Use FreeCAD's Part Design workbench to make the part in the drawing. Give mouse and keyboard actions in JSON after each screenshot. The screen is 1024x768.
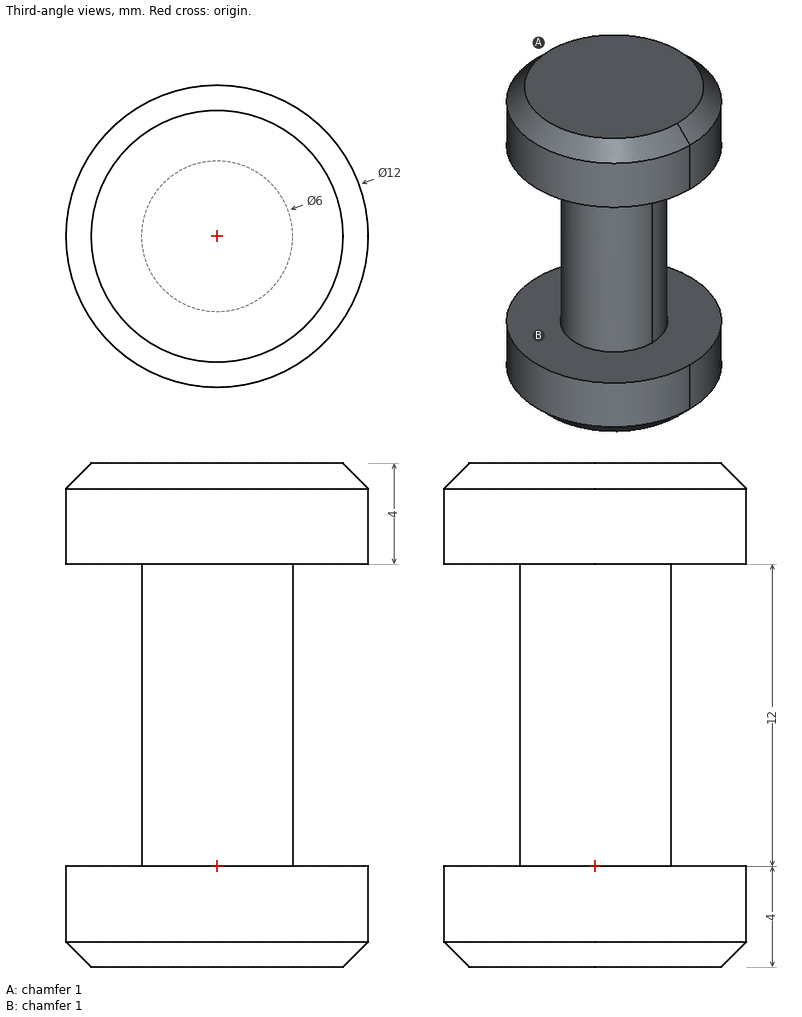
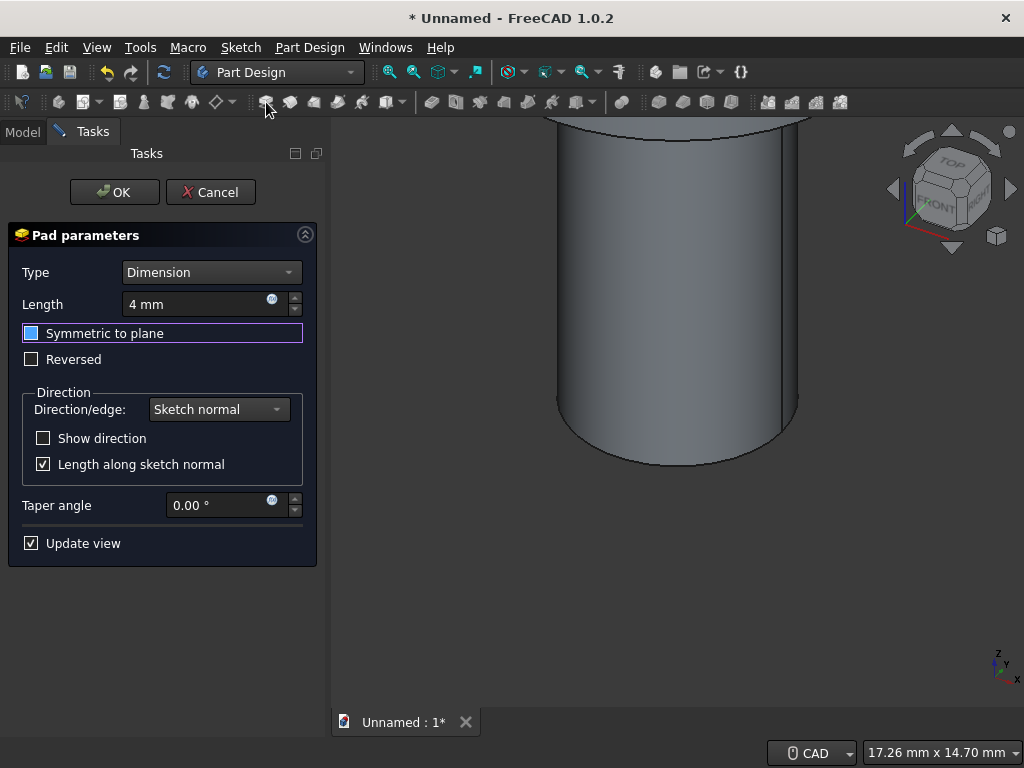
{"action": "left_click", "coordinate": [115, 192]}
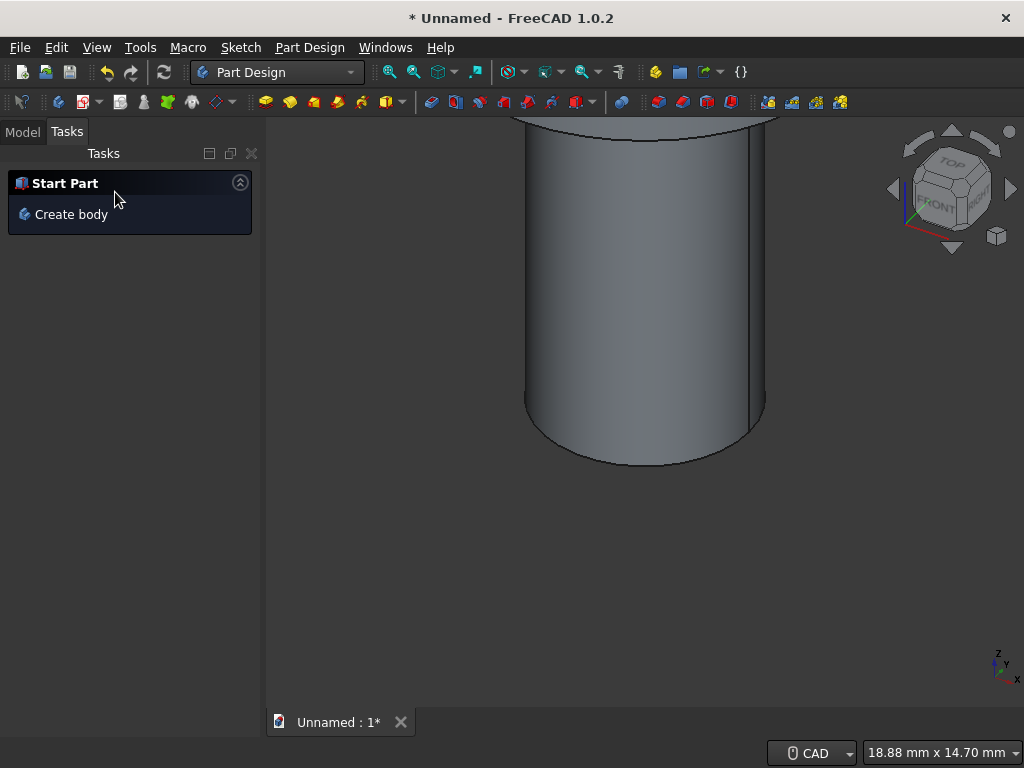
{"action": "left_click", "coordinate": [390, 72]}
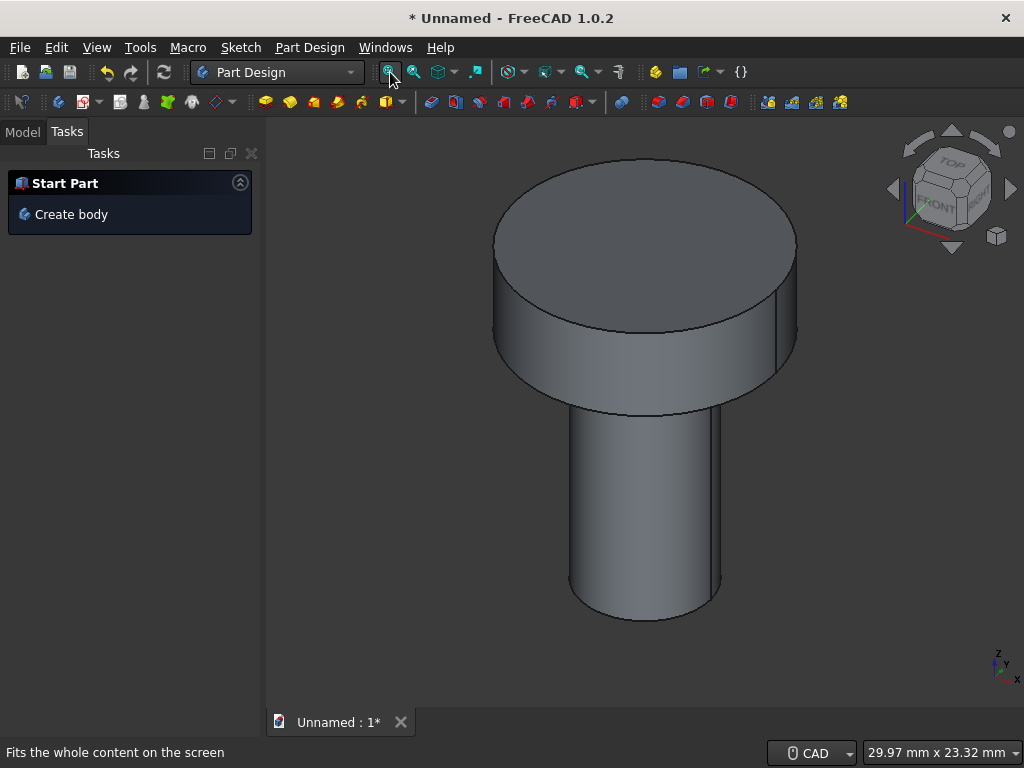
{"action": "left_click", "coordinate": [494, 254]}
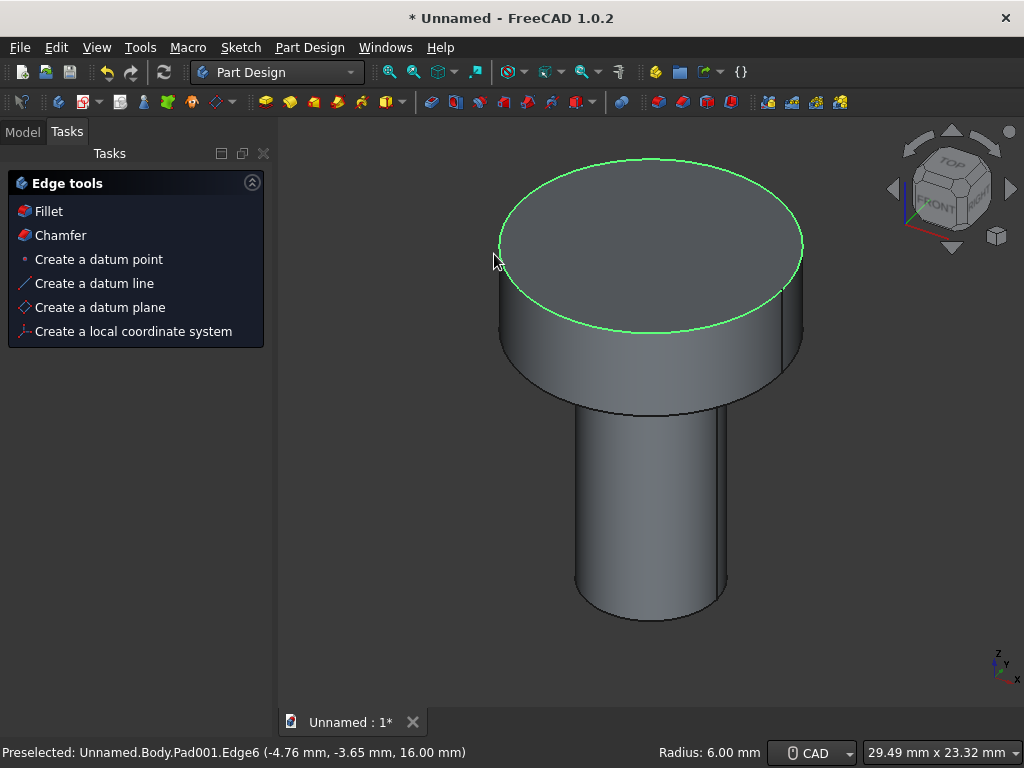
{"action": "left_click", "coordinate": [684, 102]}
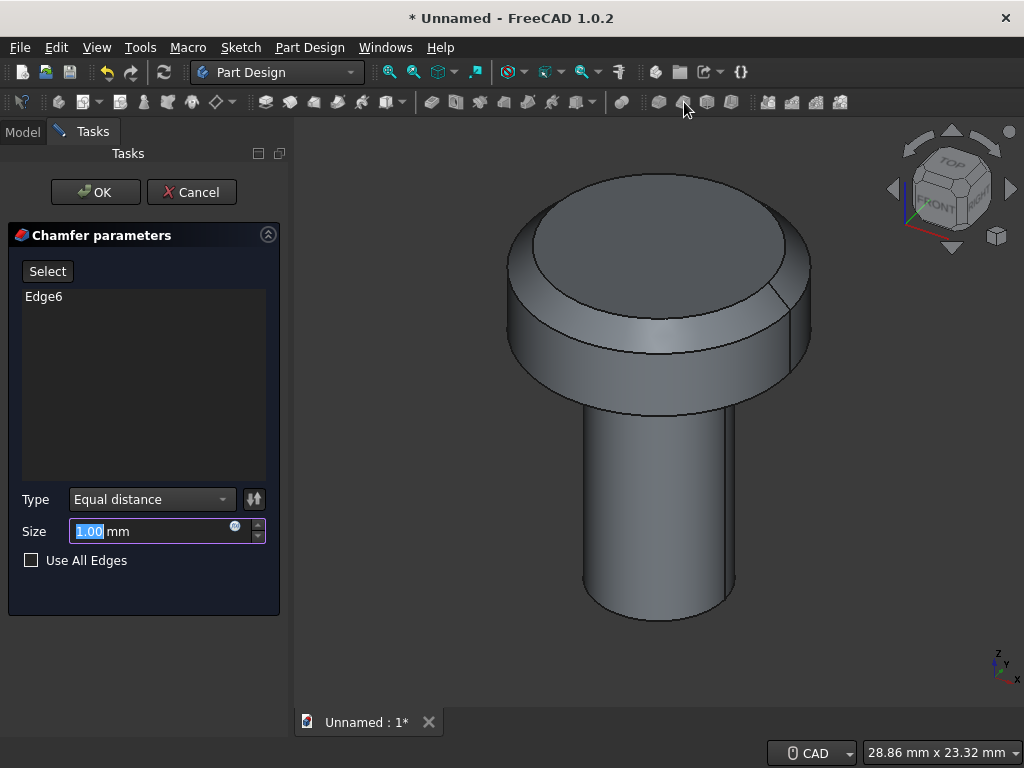
{"action": "type", "text": "1"}
{"action": "key", "text": "Tab"}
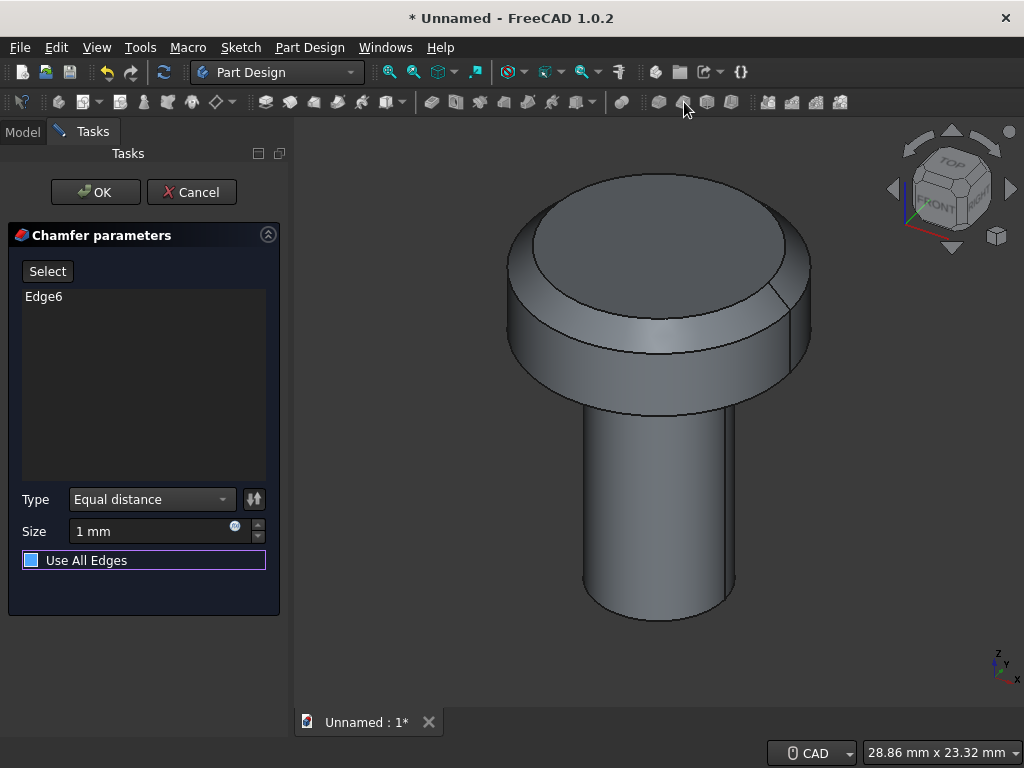
{"action": "left_click", "coordinate": [96, 192]}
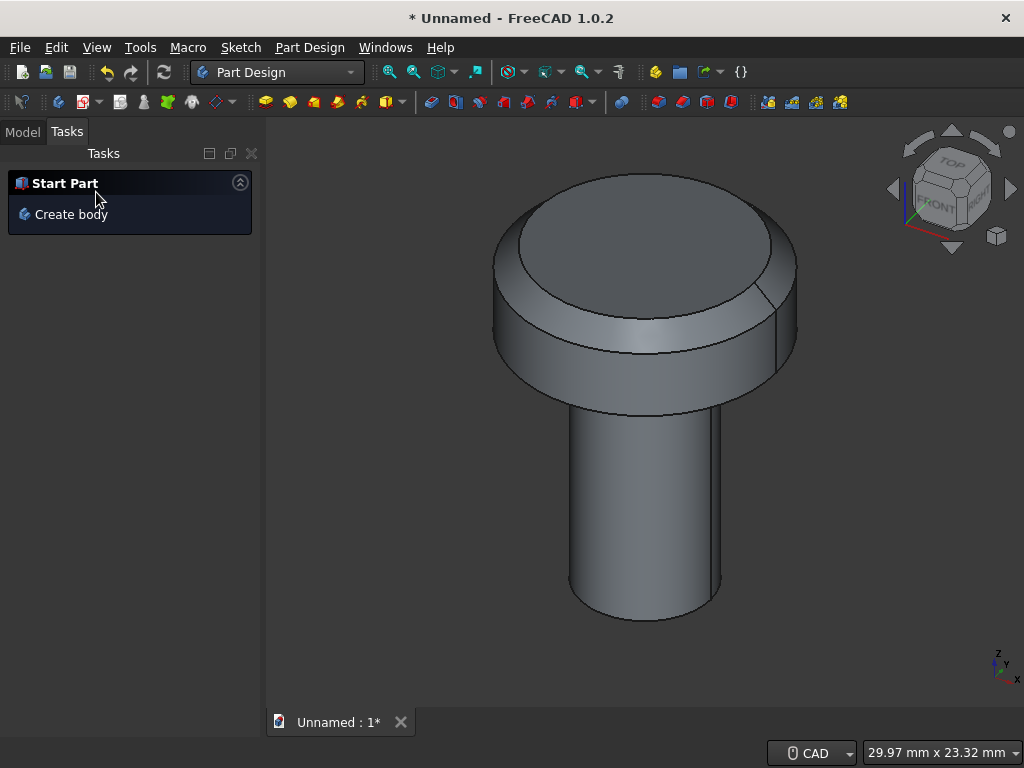
{"action": "left_click", "coordinate": [23, 131]}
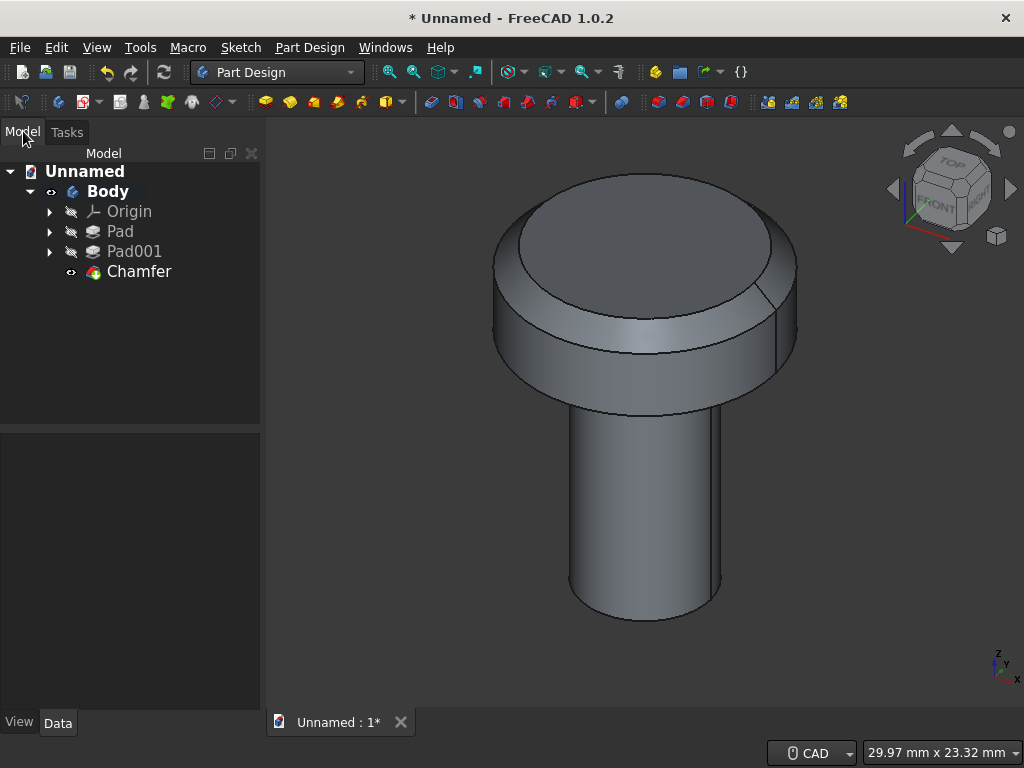
{"action": "left_click", "coordinate": [50, 212]}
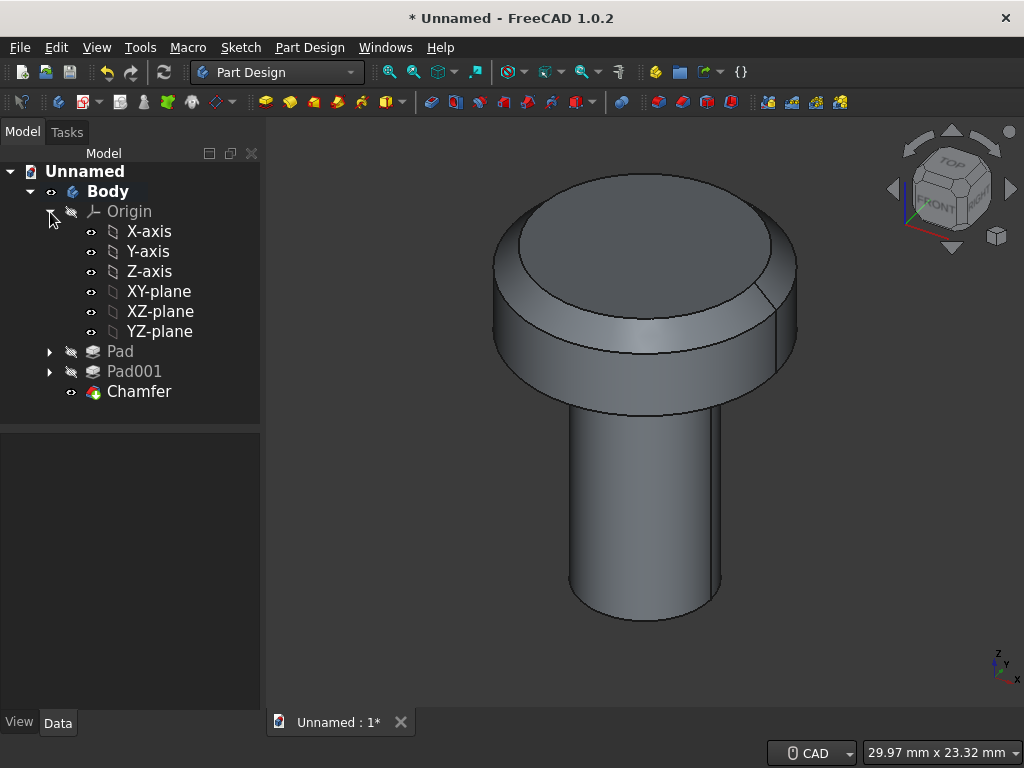
{"action": "left_click", "coordinate": [136, 292]}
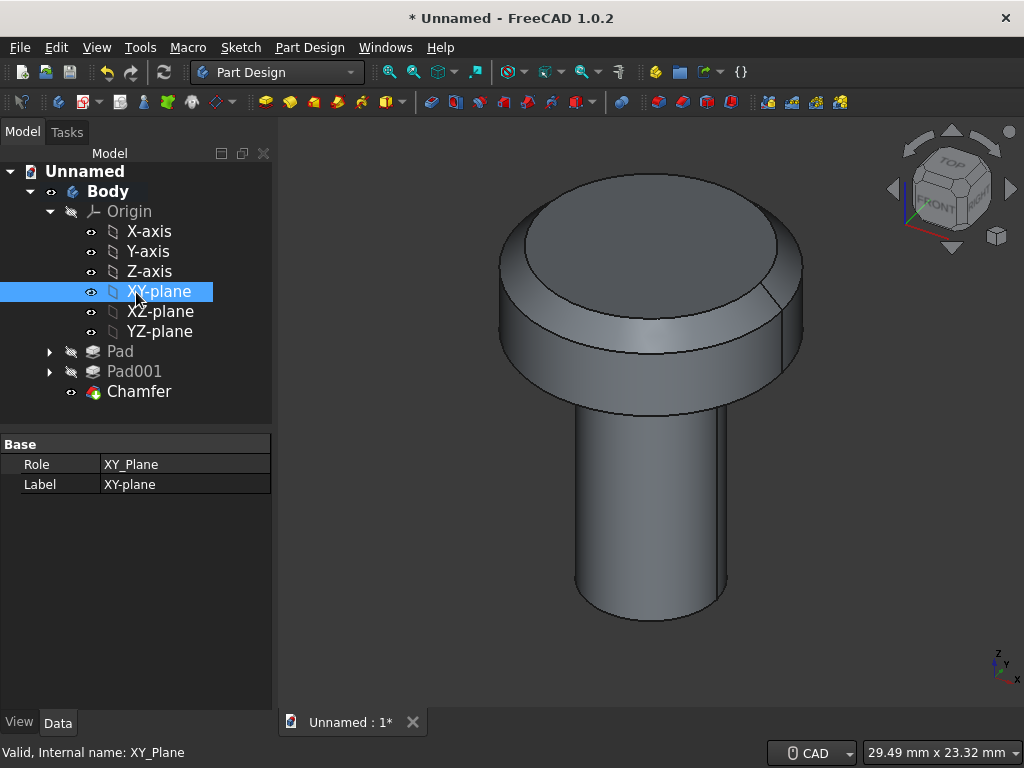
{"action": "left_click", "coordinate": [216, 102]}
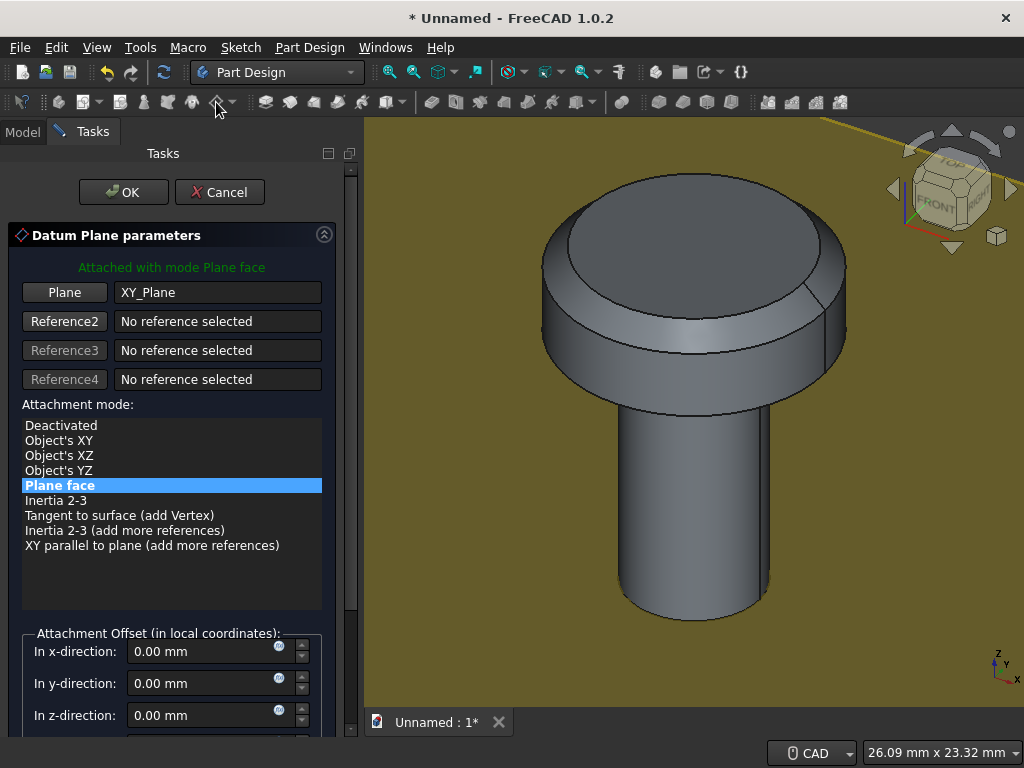
{"action": "triple_click", "coordinate": [210, 715]}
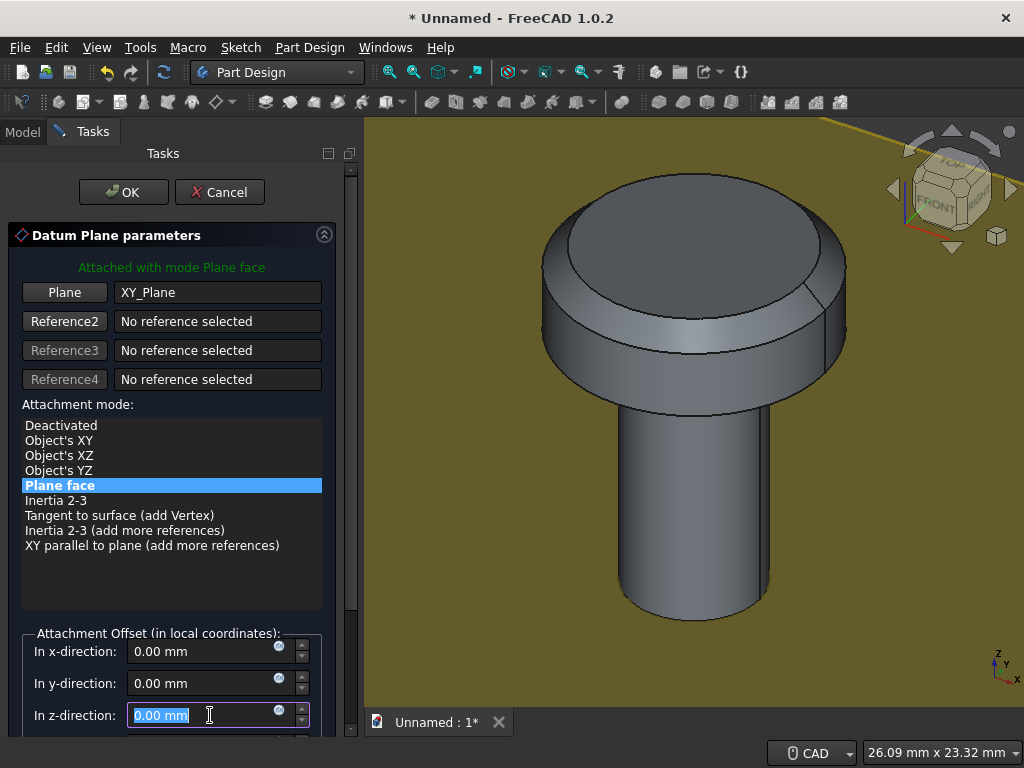
{"action": "type", "text": "-4"}
{"action": "key", "text": "Tab"}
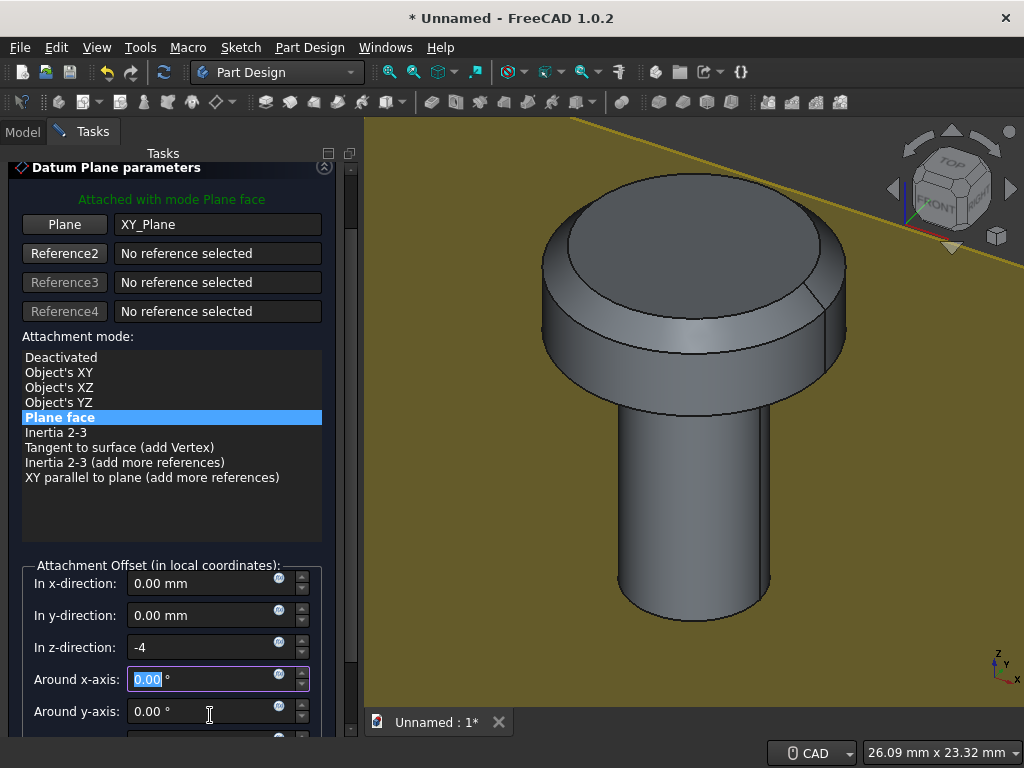
{"action": "scroll", "coordinate": [351, 450], "scroll_direction": "up", "scroll_amount": 2}